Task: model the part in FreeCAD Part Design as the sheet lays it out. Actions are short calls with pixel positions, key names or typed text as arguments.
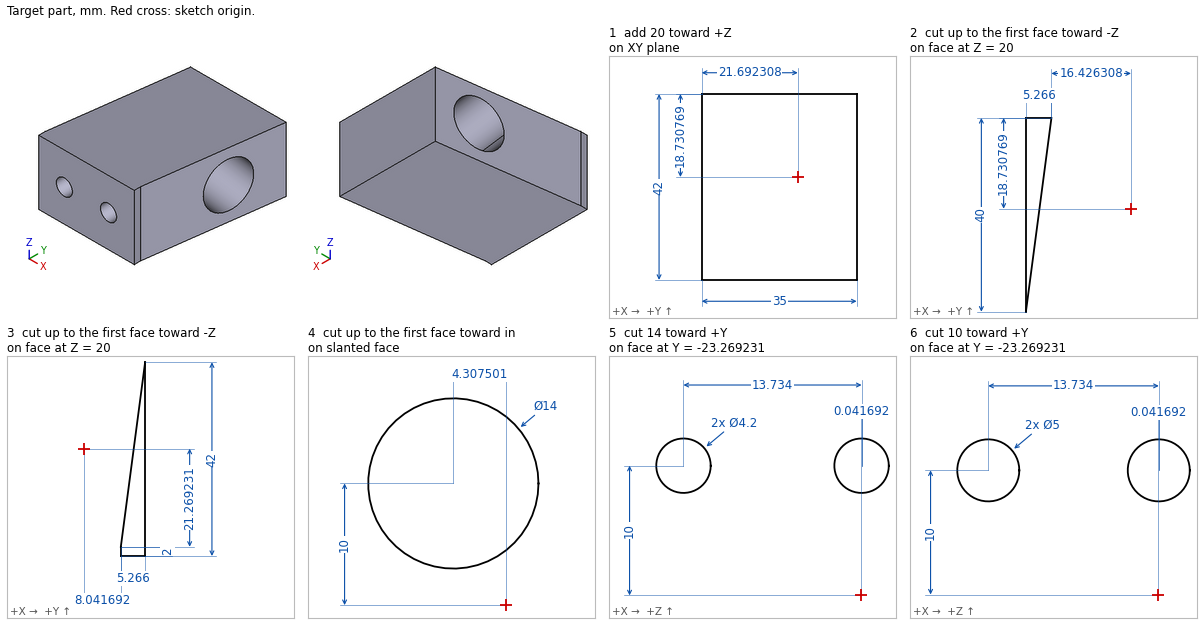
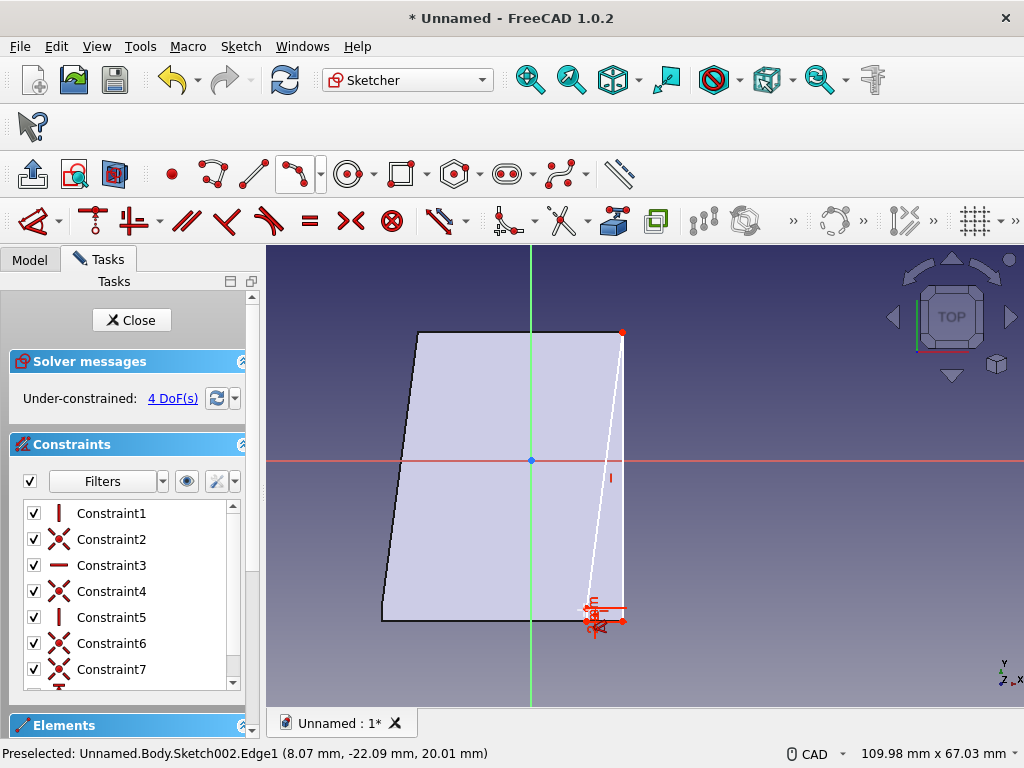
click(623, 535)
click(657, 477)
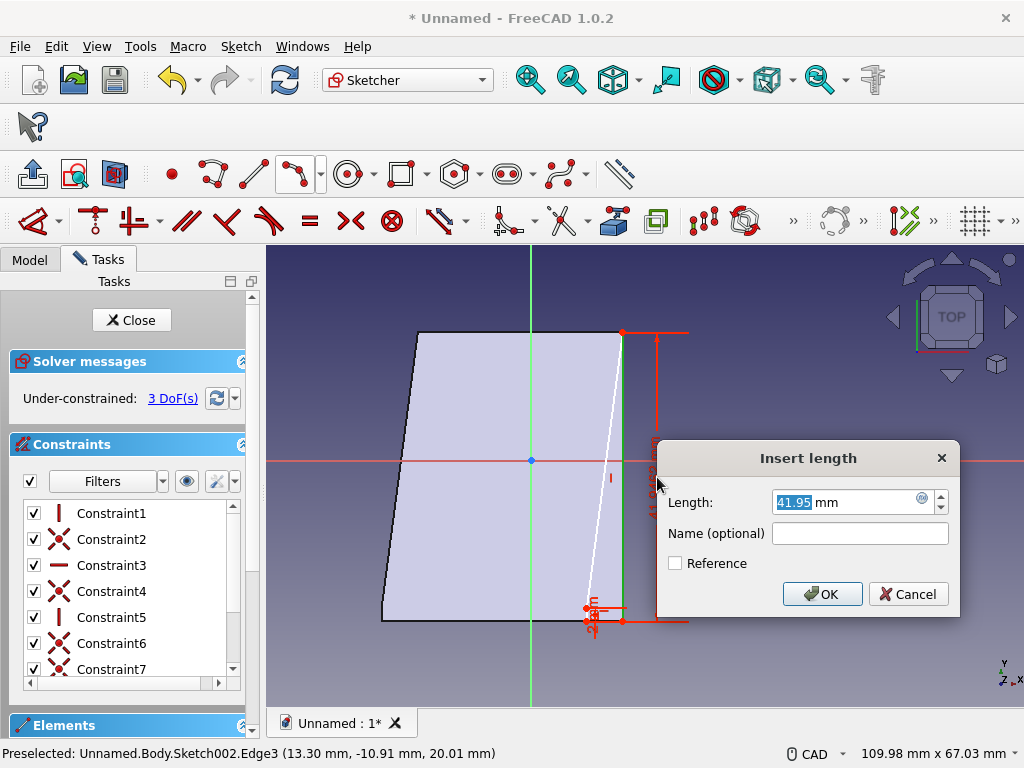
text(42)
key(Return)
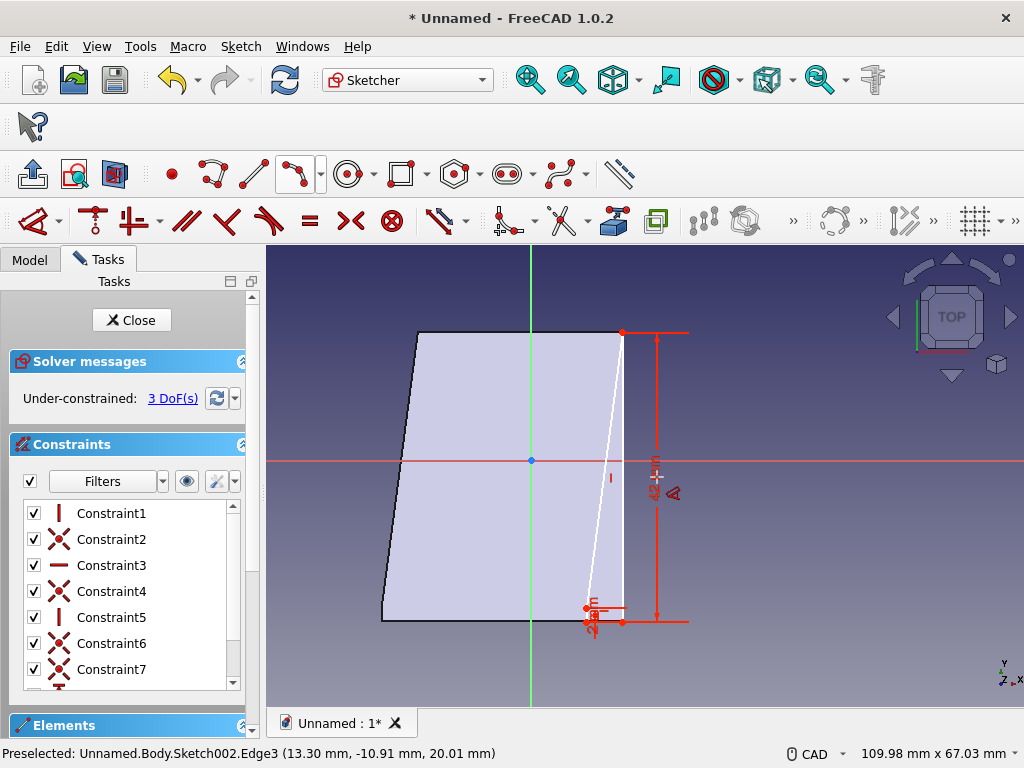
scroll(598, 622, up, 2)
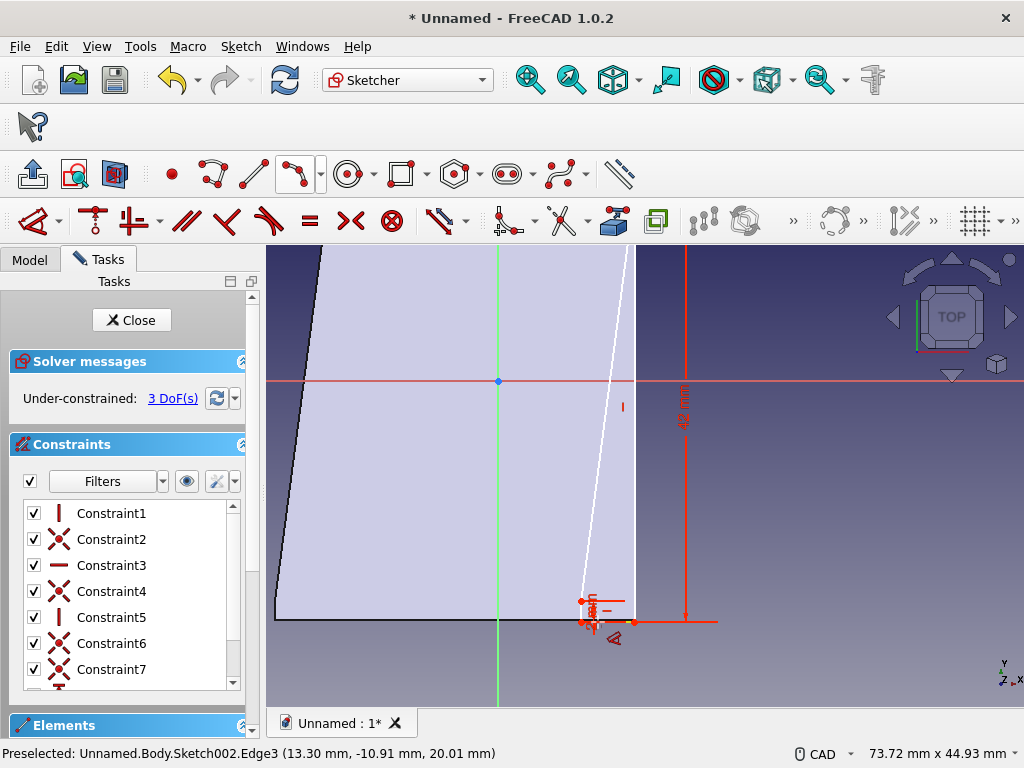
click(597, 622)
click(608, 656)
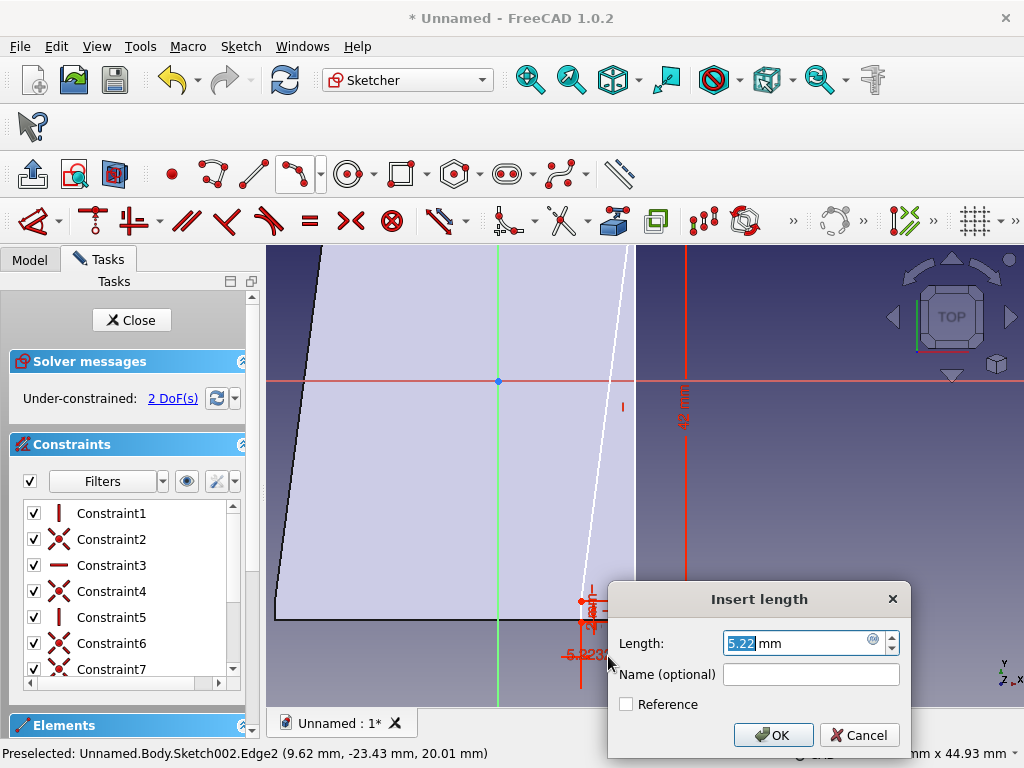
text(5.266)
key(Return)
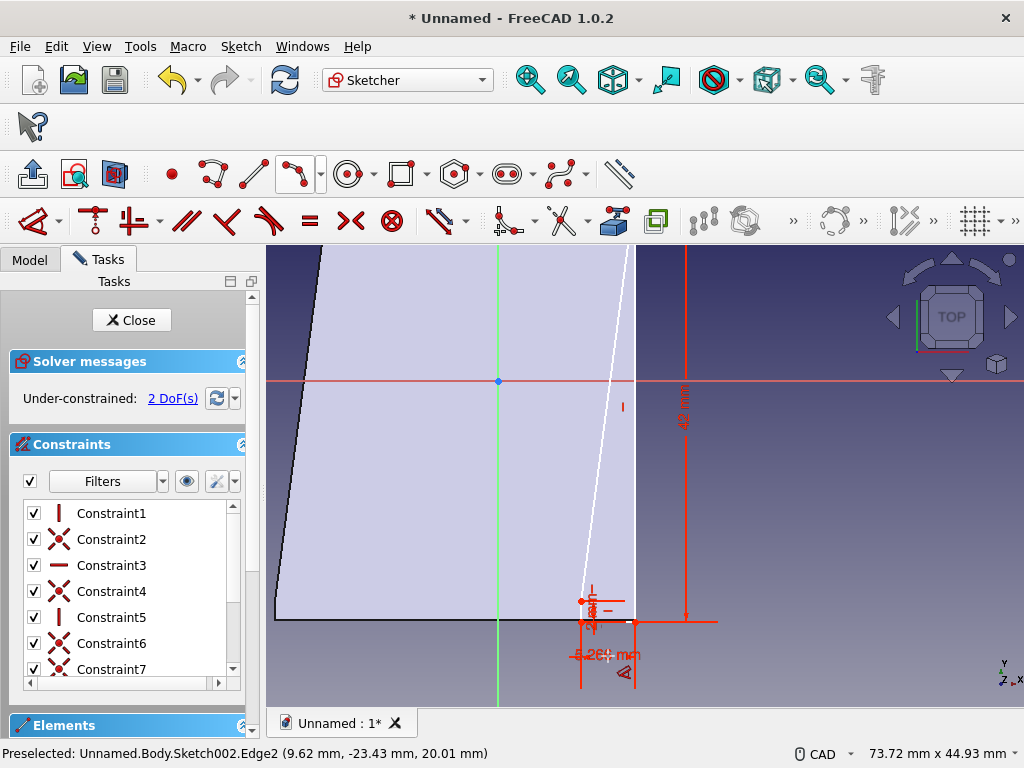
click(581, 601)
click(540, 635)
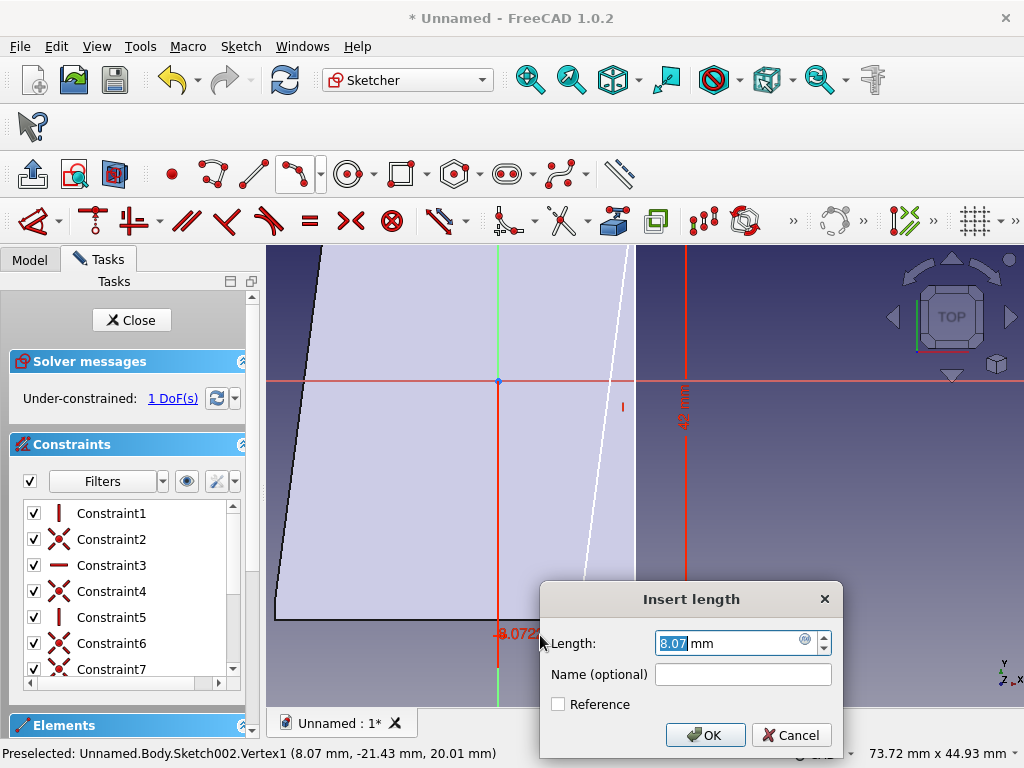
text(8.041692)
key(Return)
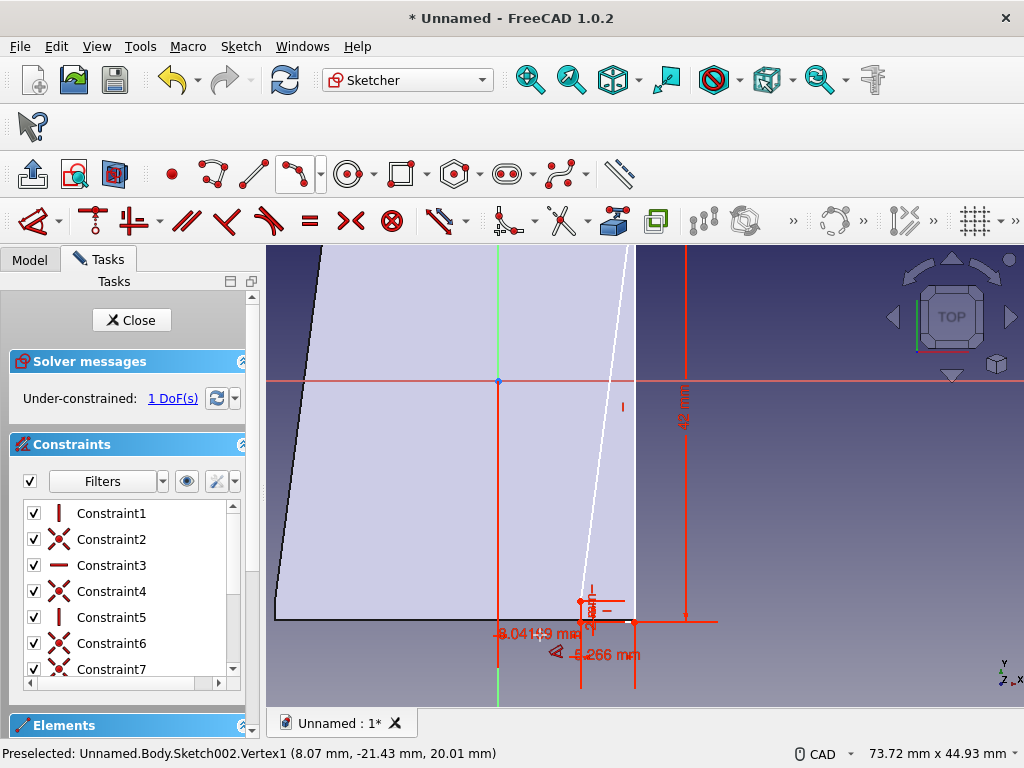
click(581, 601)
click(464, 491)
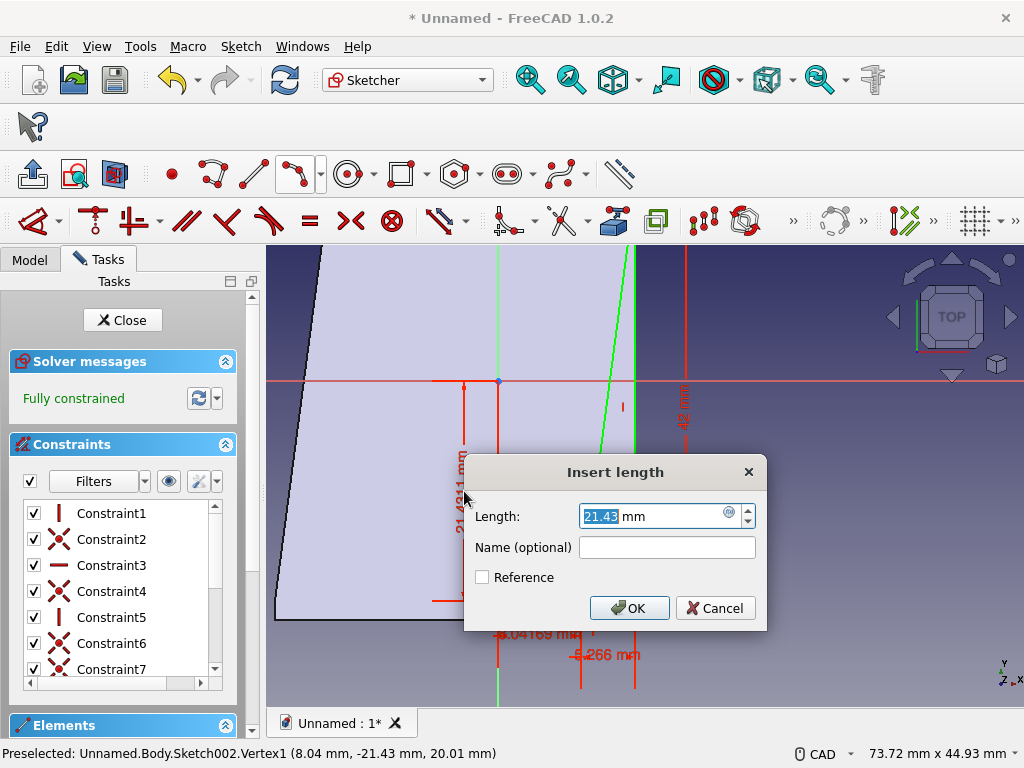
text(21.269231)
key(Return)
key(Escape)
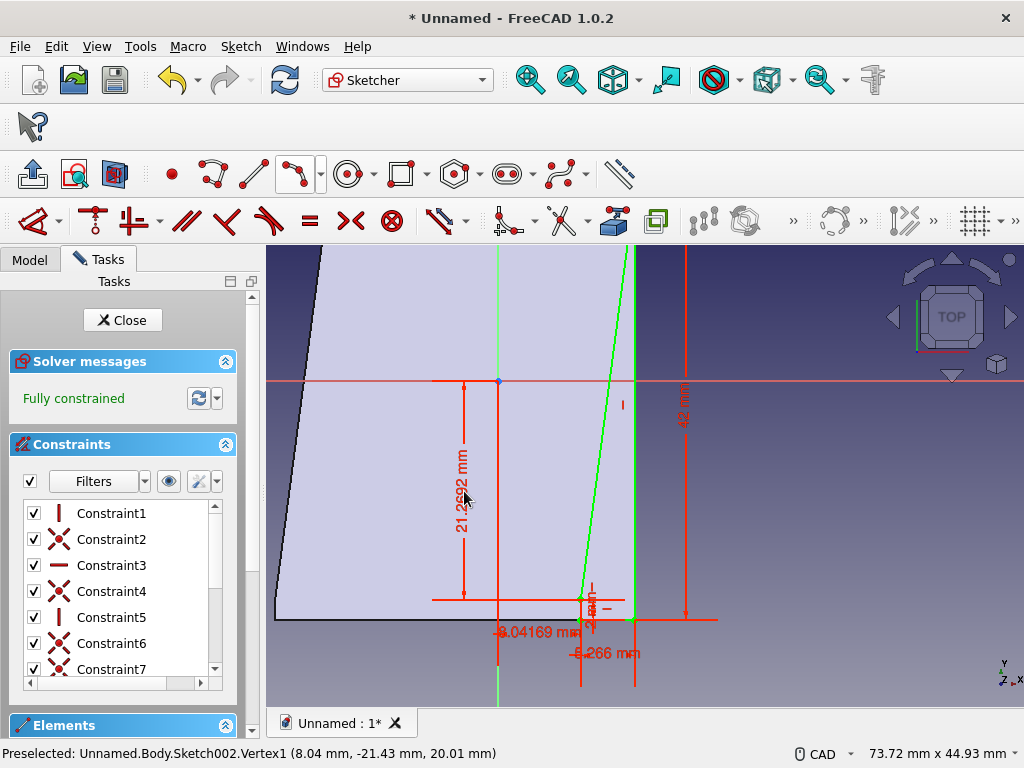
click(123, 320)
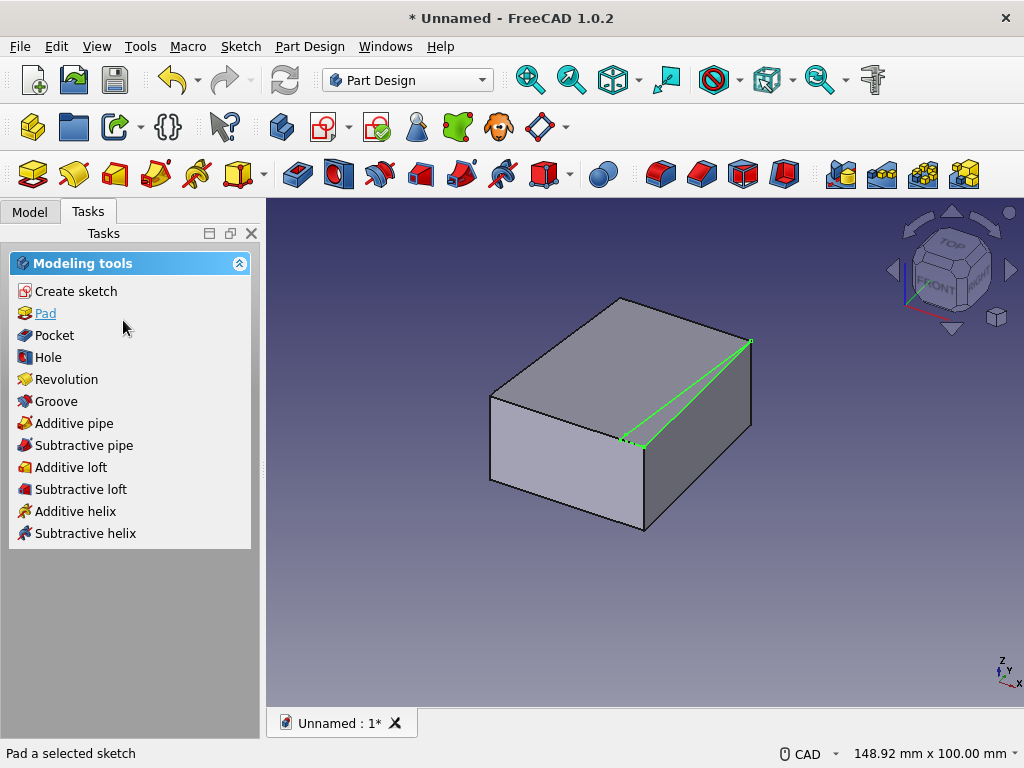
click(298, 174)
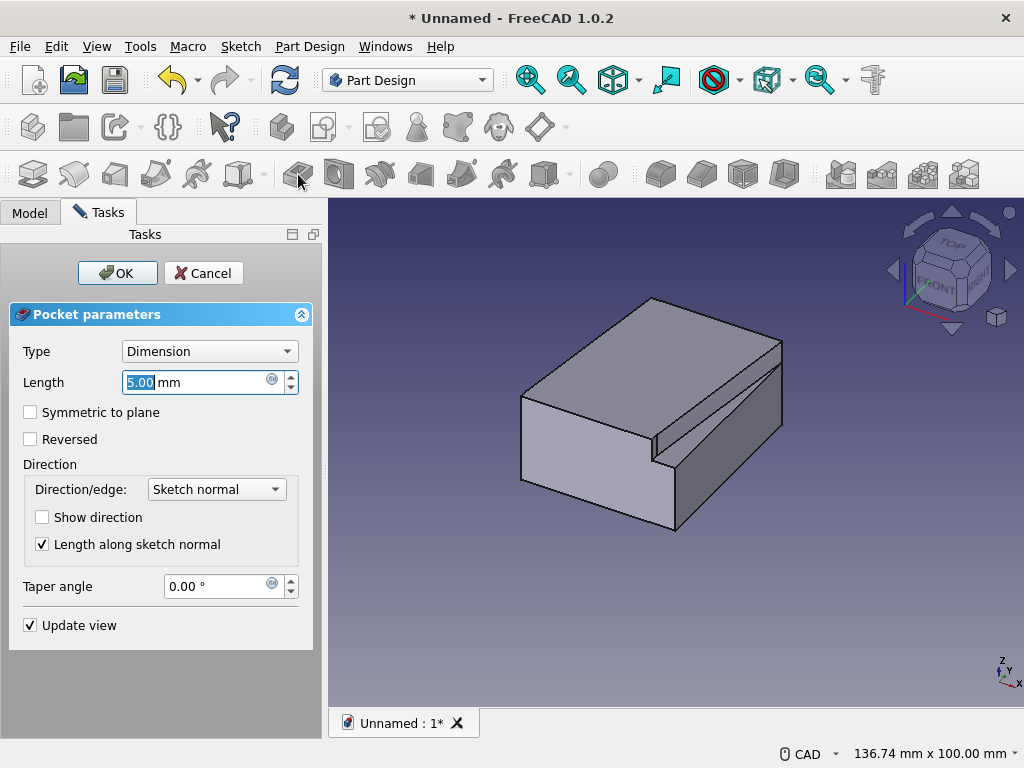
click(210, 352)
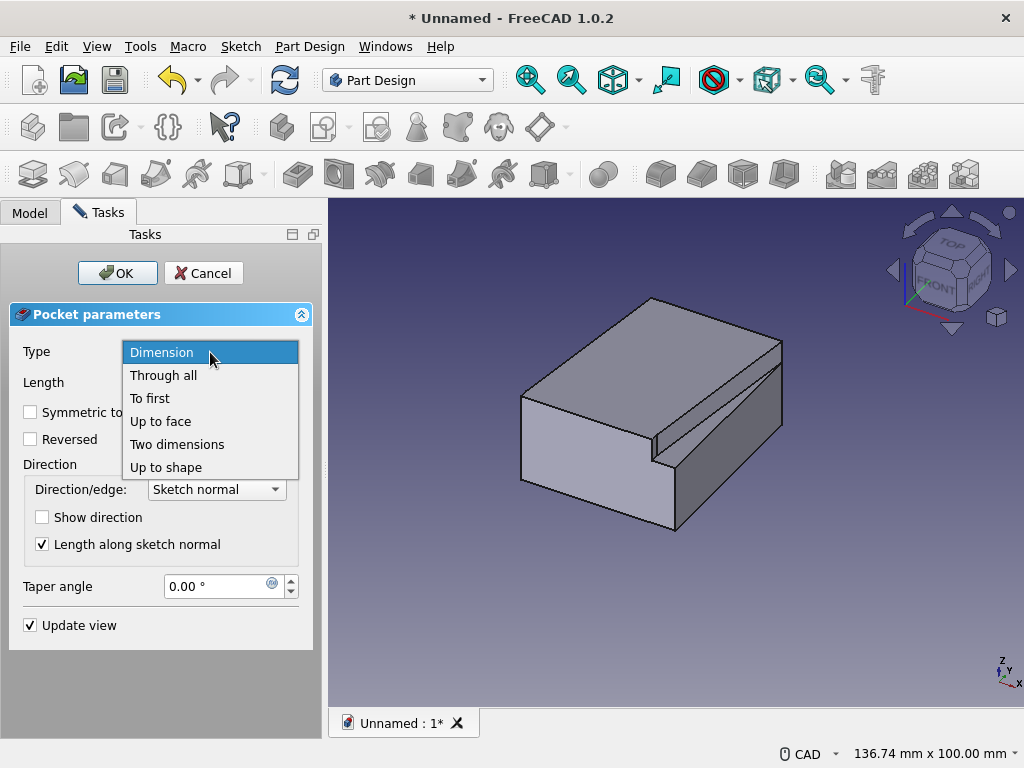
click(208, 398)